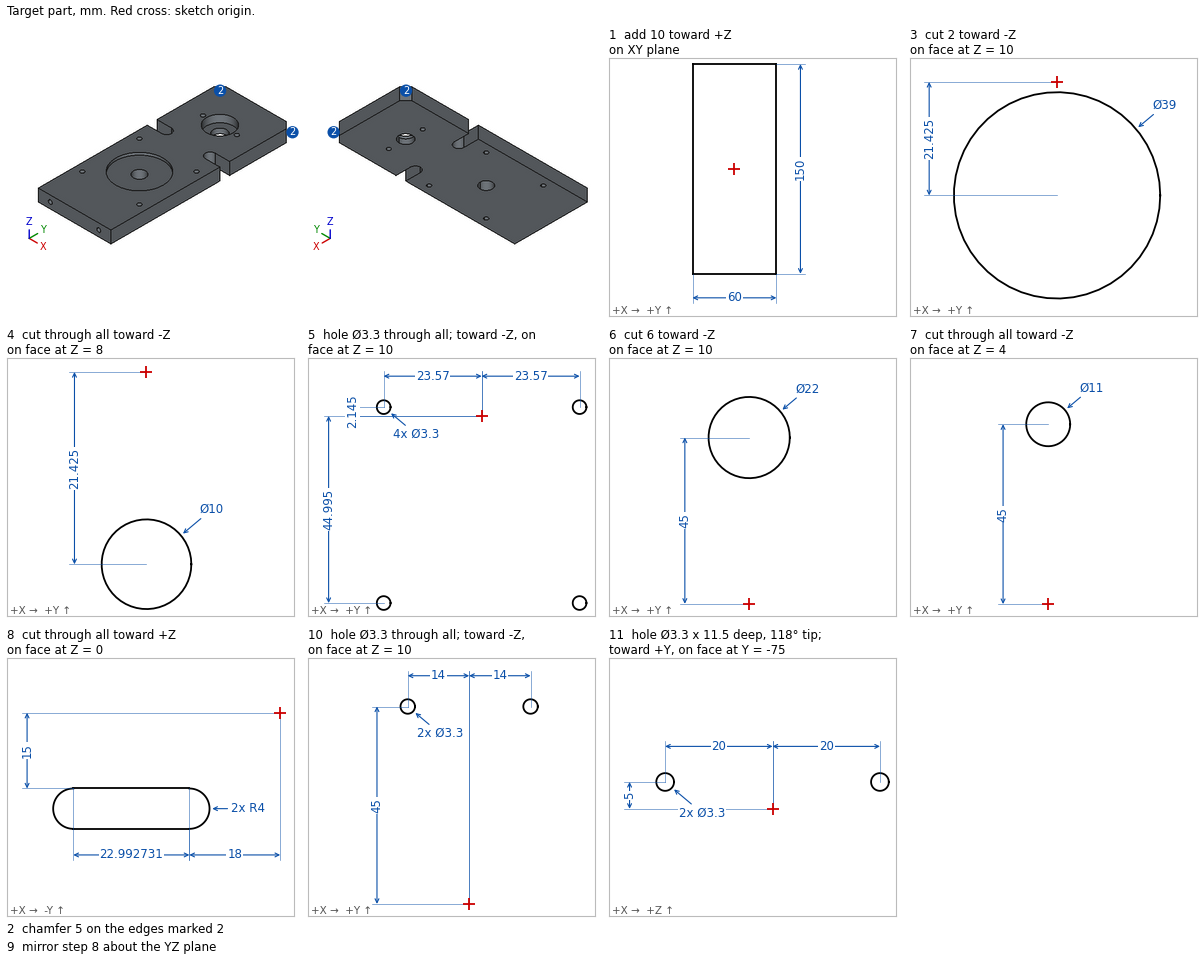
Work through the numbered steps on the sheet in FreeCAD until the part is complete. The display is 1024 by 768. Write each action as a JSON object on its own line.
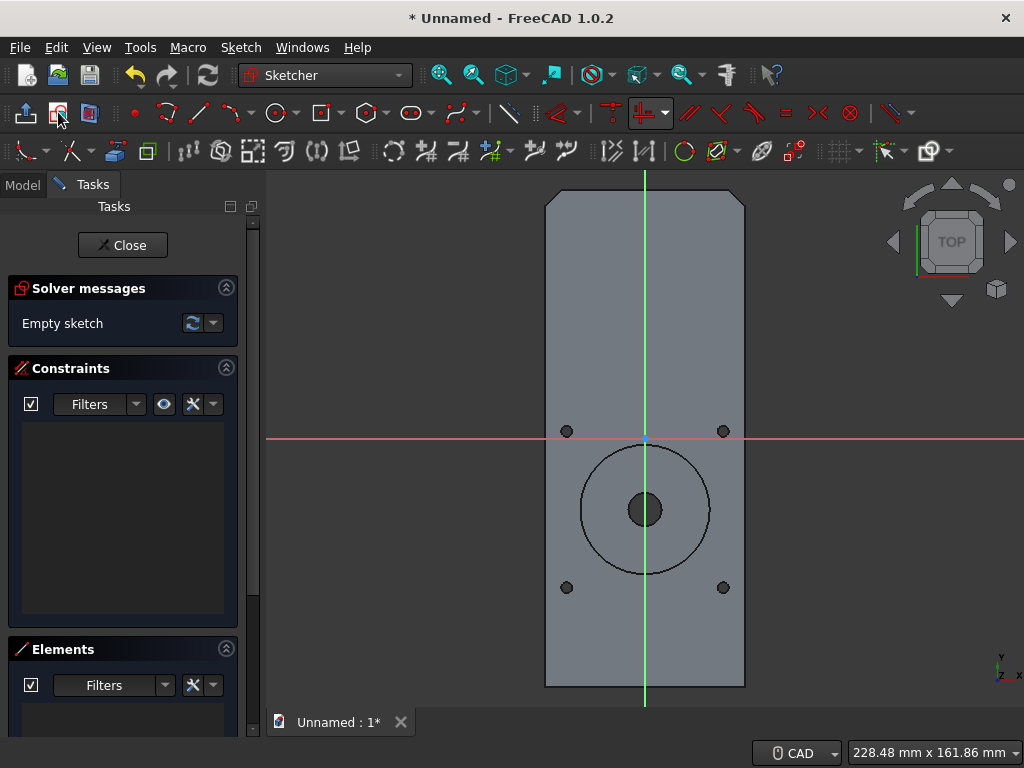
{"action": "scroll", "coordinate": [662, 251], "scroll_direction": "up", "scroll_amount": 8}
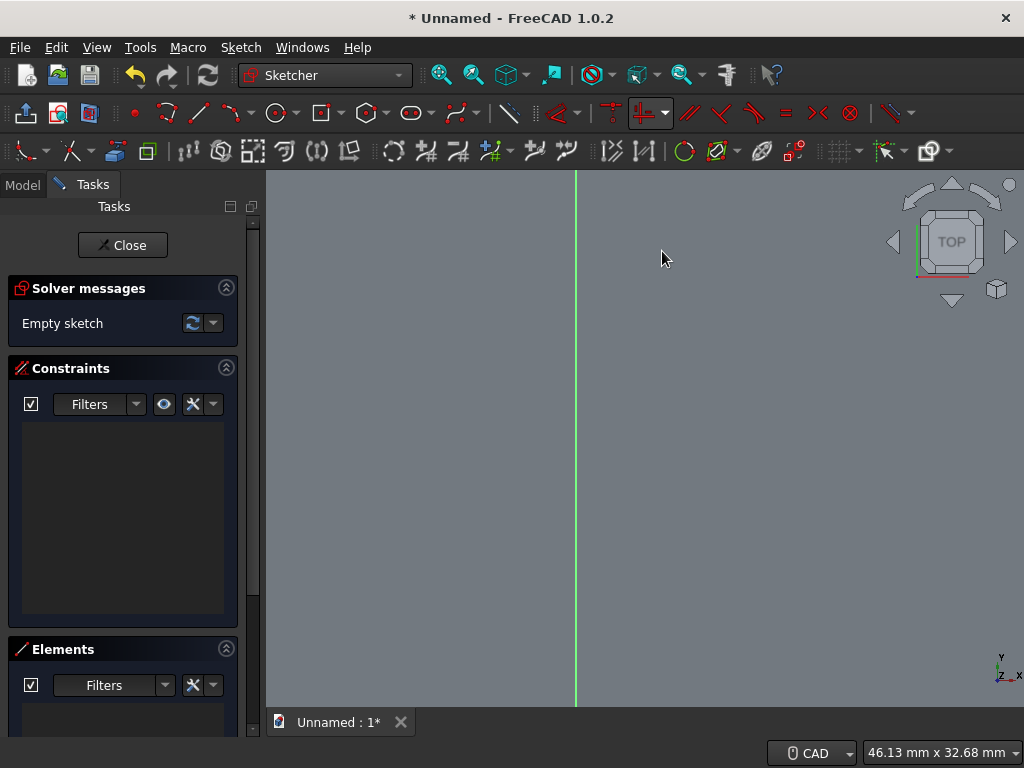
{"action": "key", "text": "g c"}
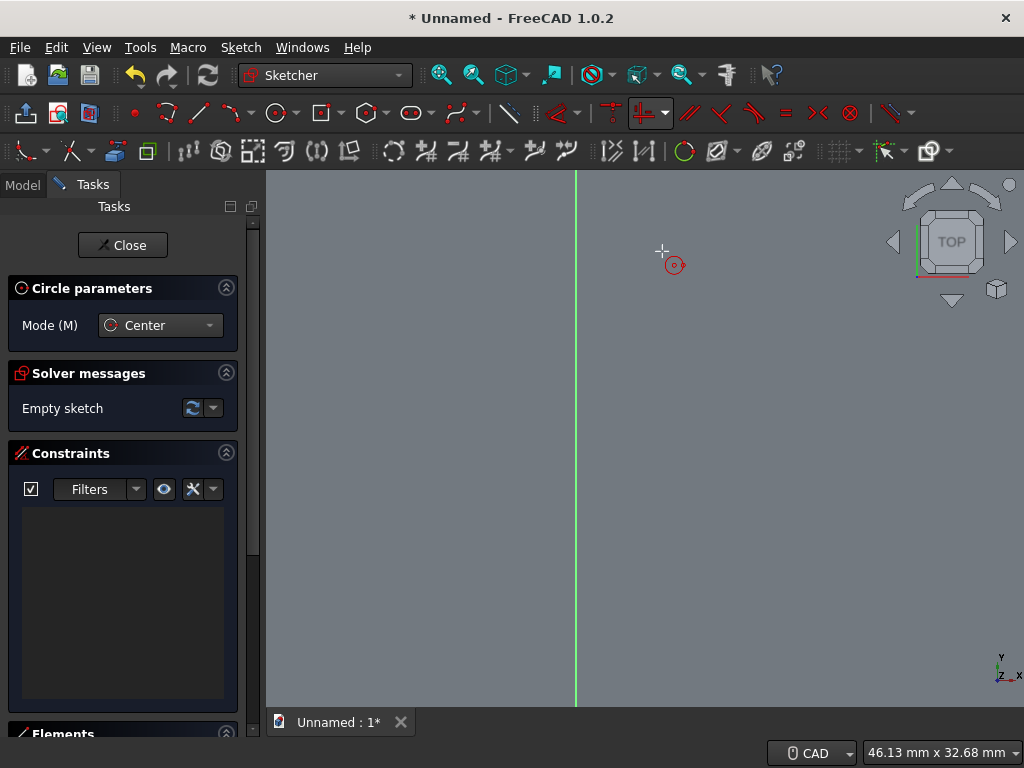
{"action": "left_click", "coordinate": [576, 440]}
{"action": "left_click", "coordinate": [704, 312]}
{"action": "key", "text": "Escape"}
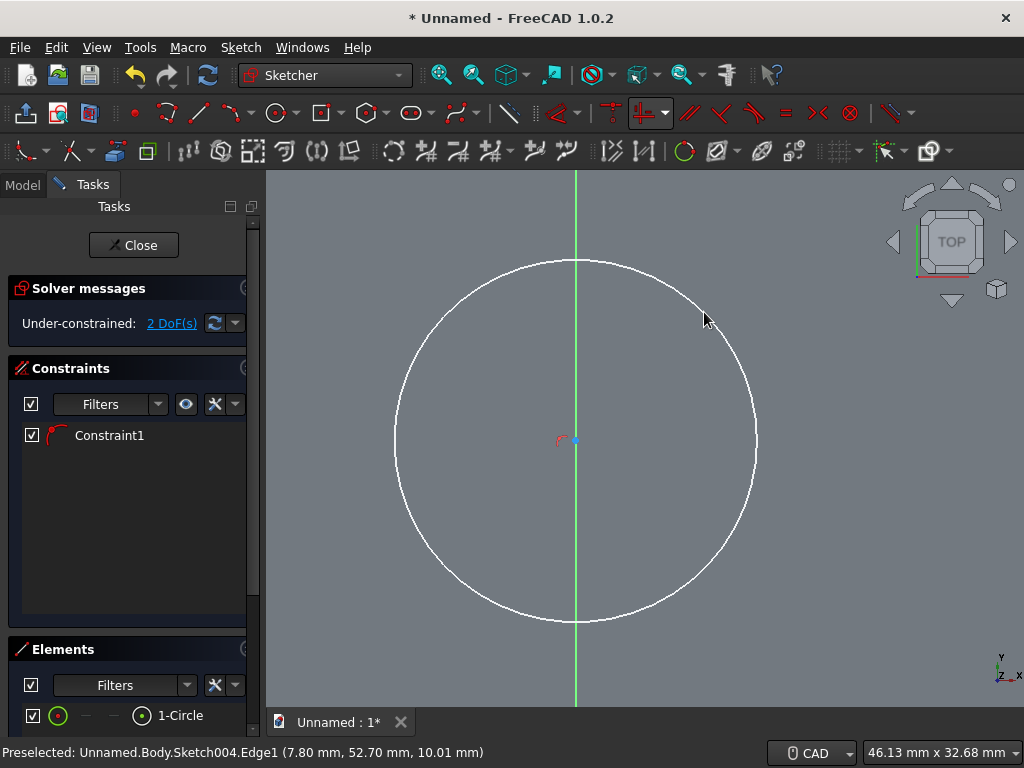
{"action": "left_click", "coordinate": [556, 114]}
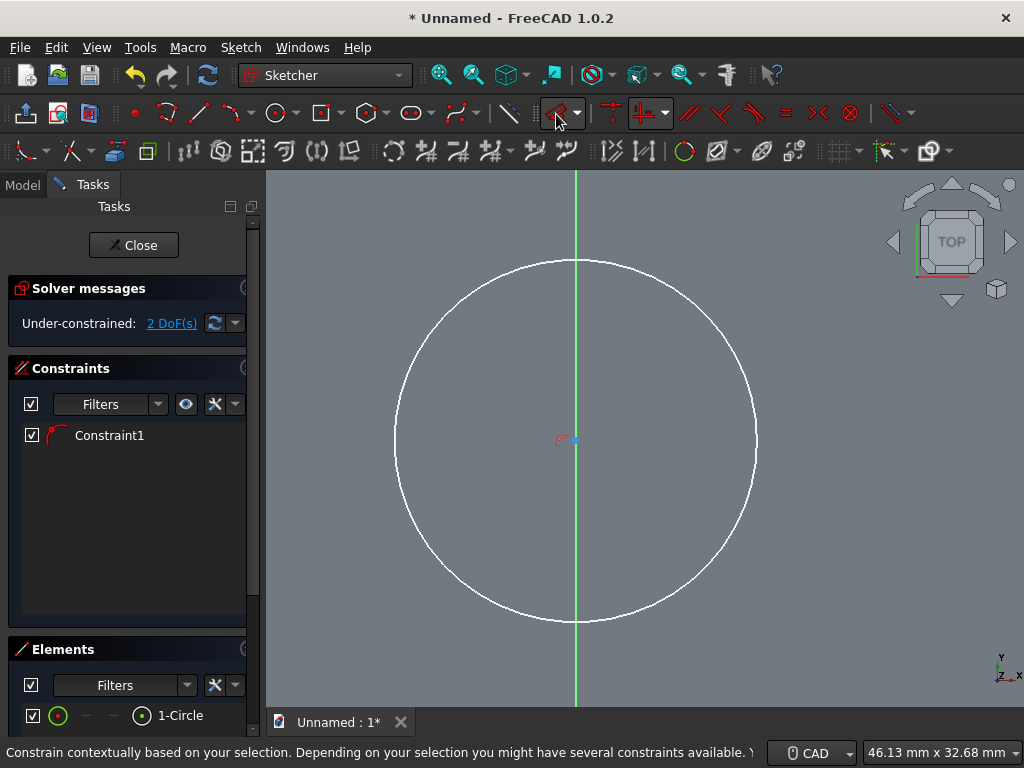
{"action": "left_click", "coordinate": [703, 312]}
{"action": "left_click", "coordinate": [725, 289]}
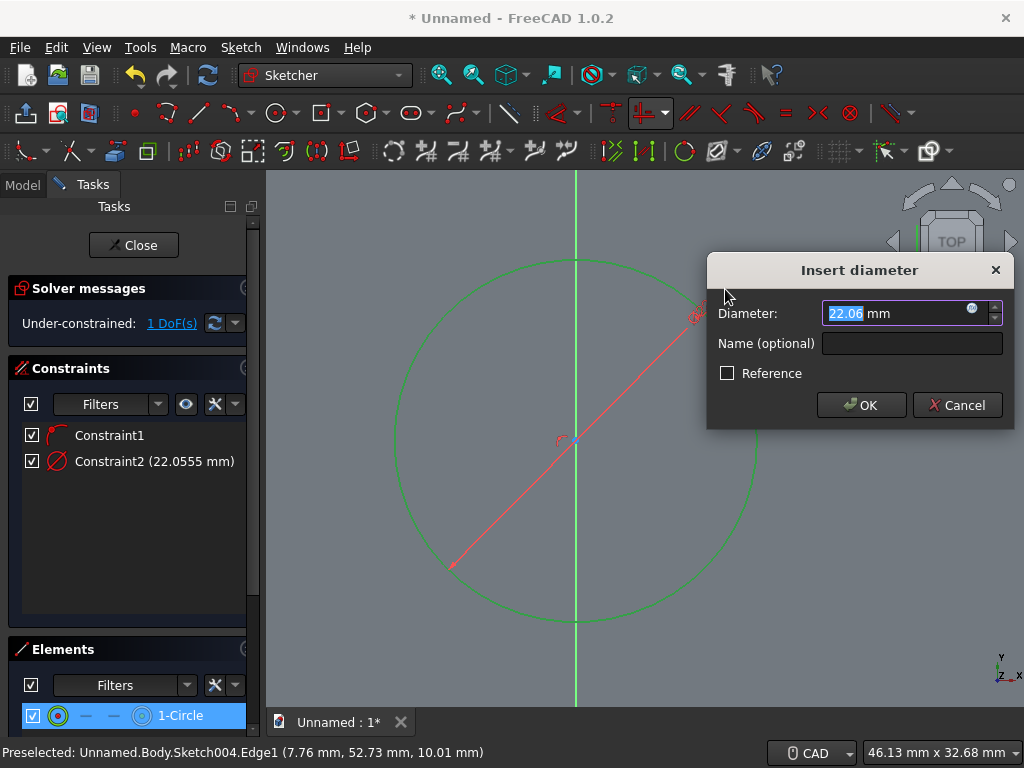
{"action": "type", "text": "22"}
{"action": "key", "text": "Return"}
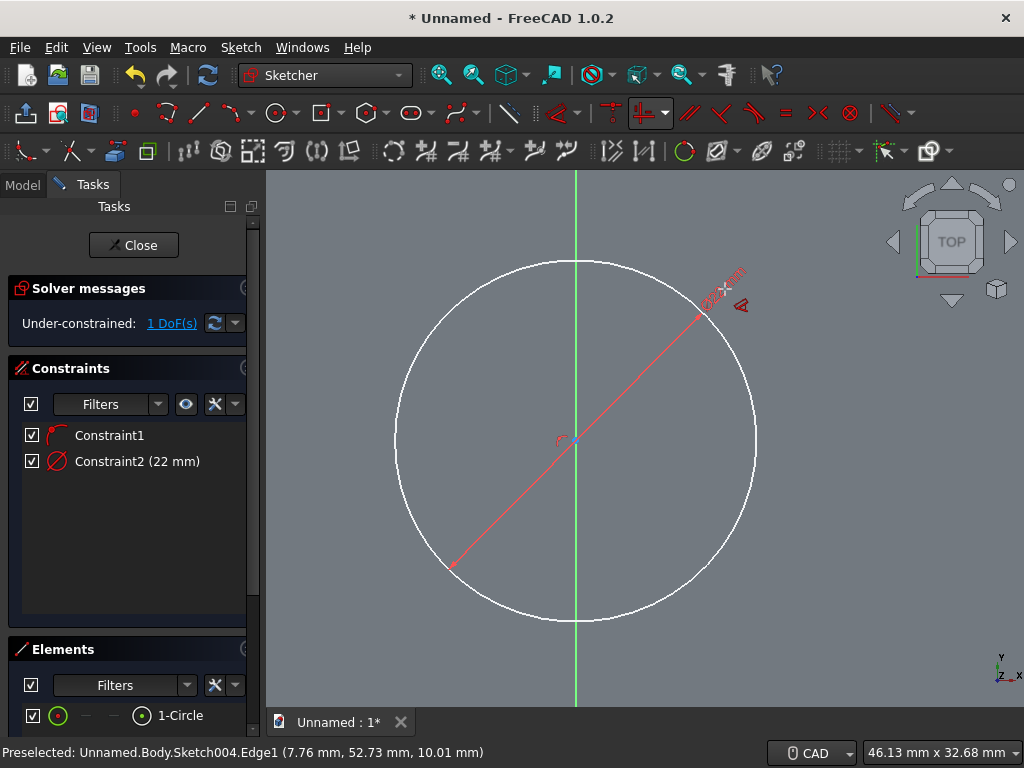
{"action": "left_click", "coordinate": [576, 441]}
{"action": "left_click", "coordinate": [610, 560]}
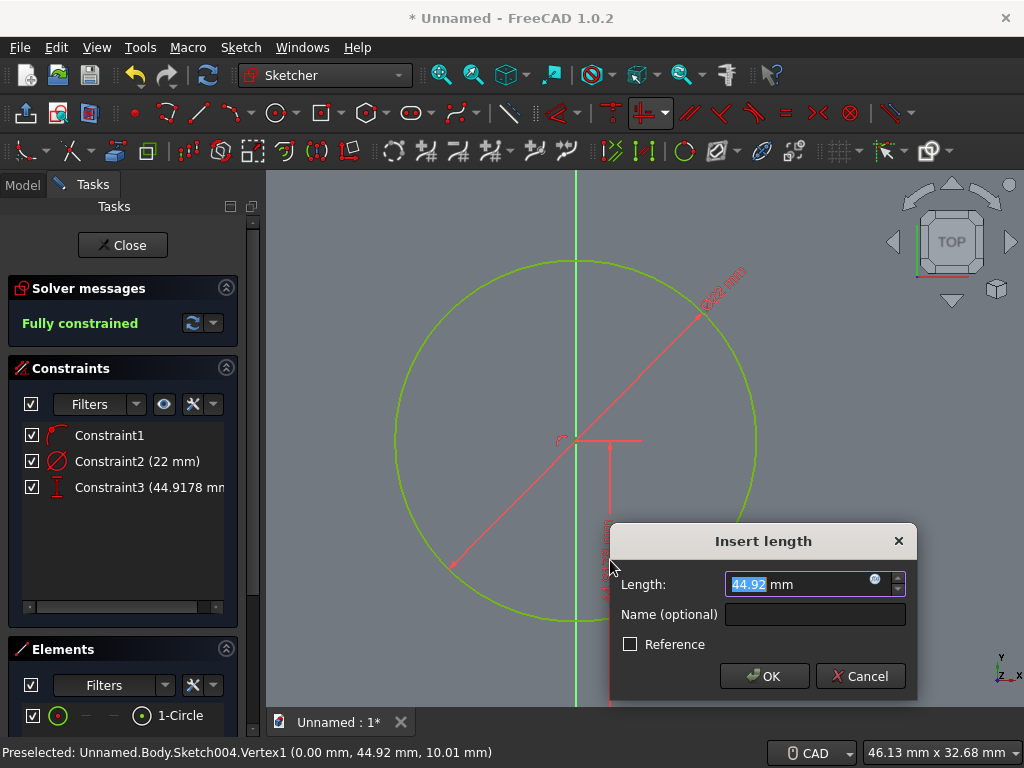
{"action": "type", "text": "45"}
{"action": "key", "text": "Return"}
{"action": "key", "text": "Escape"}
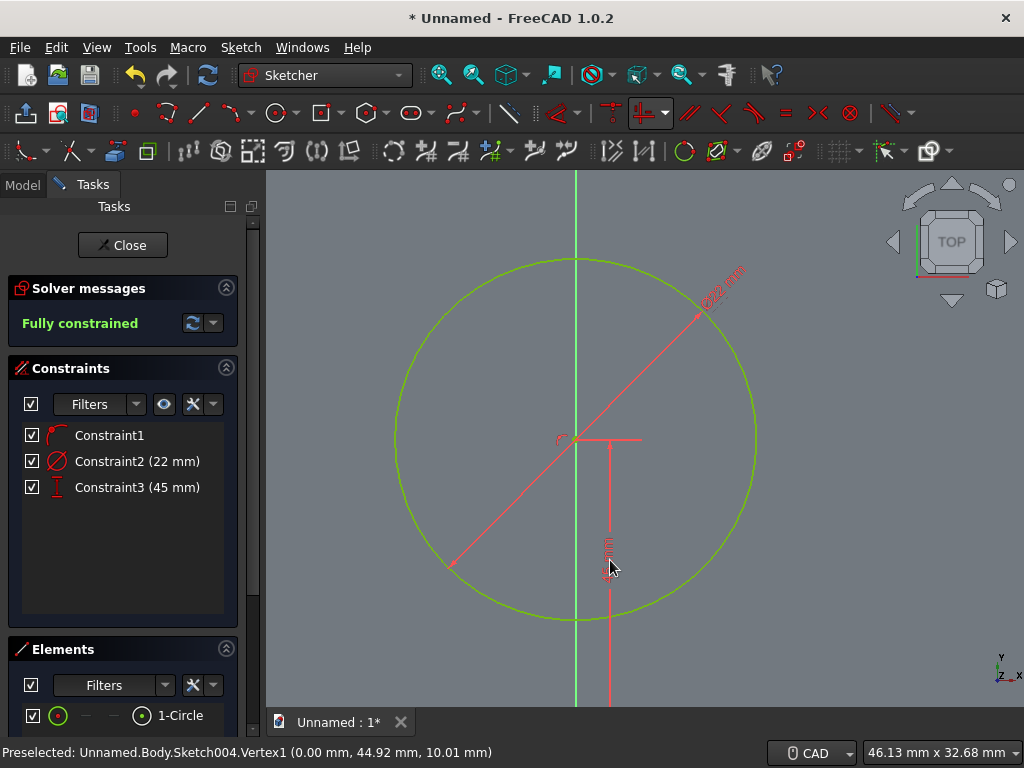
{"action": "left_click", "coordinate": [123, 245]}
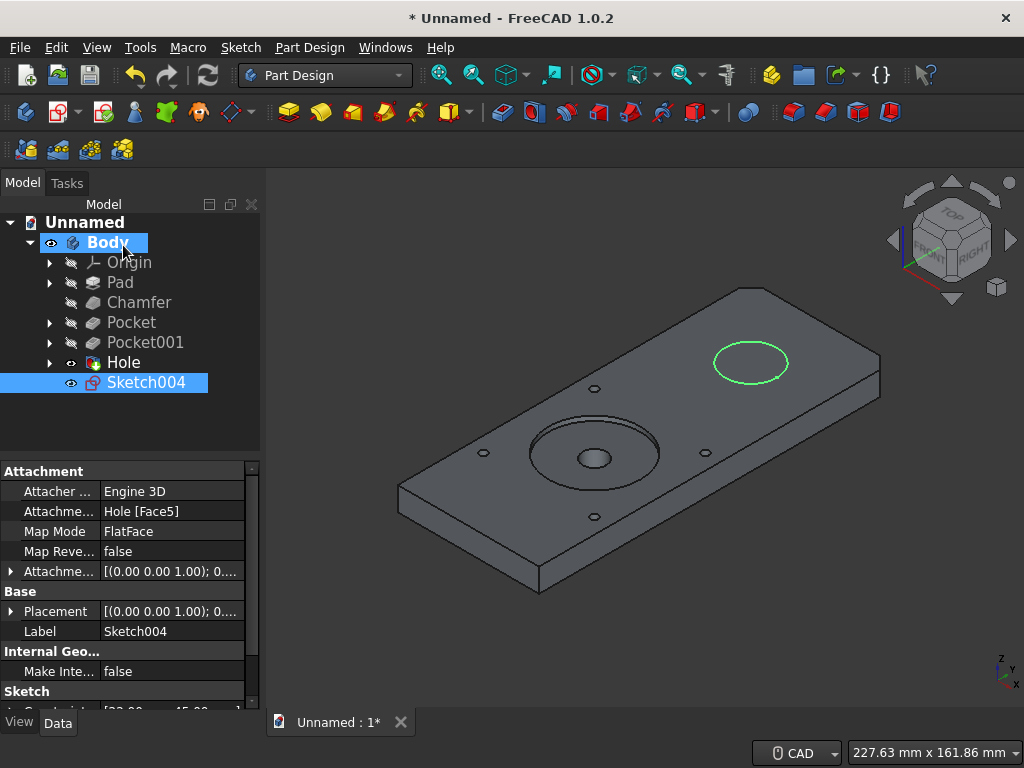
{"action": "left_click", "coordinate": [504, 112]}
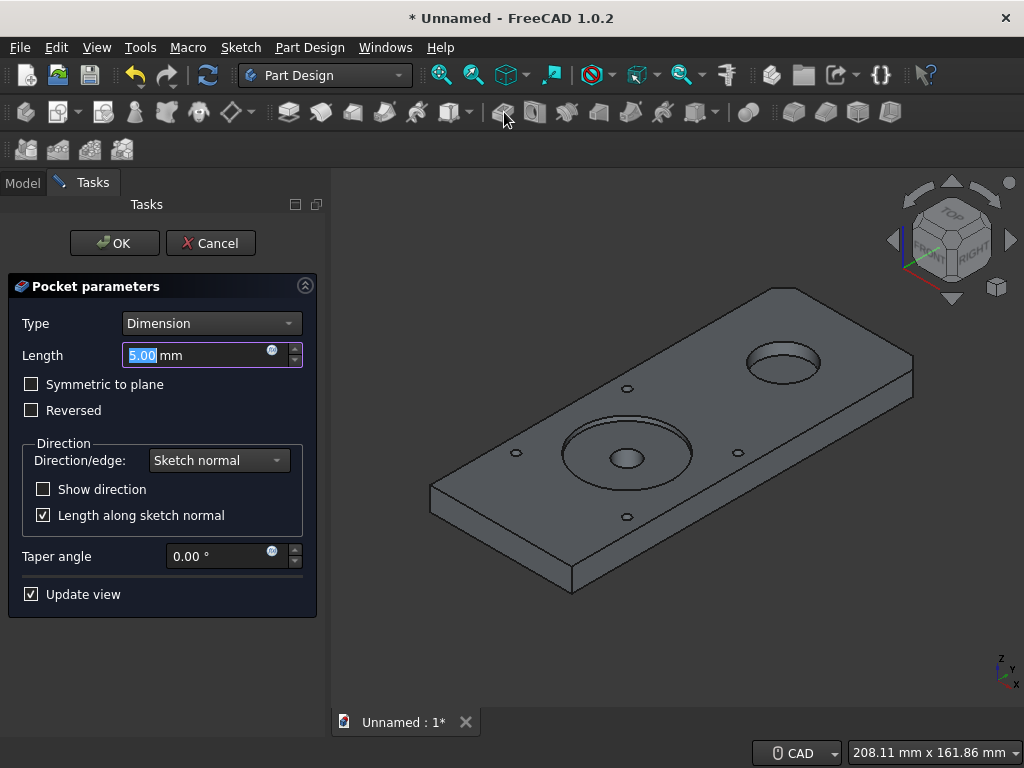
{"action": "type", "text": "6"}
{"action": "key", "text": "Tab"}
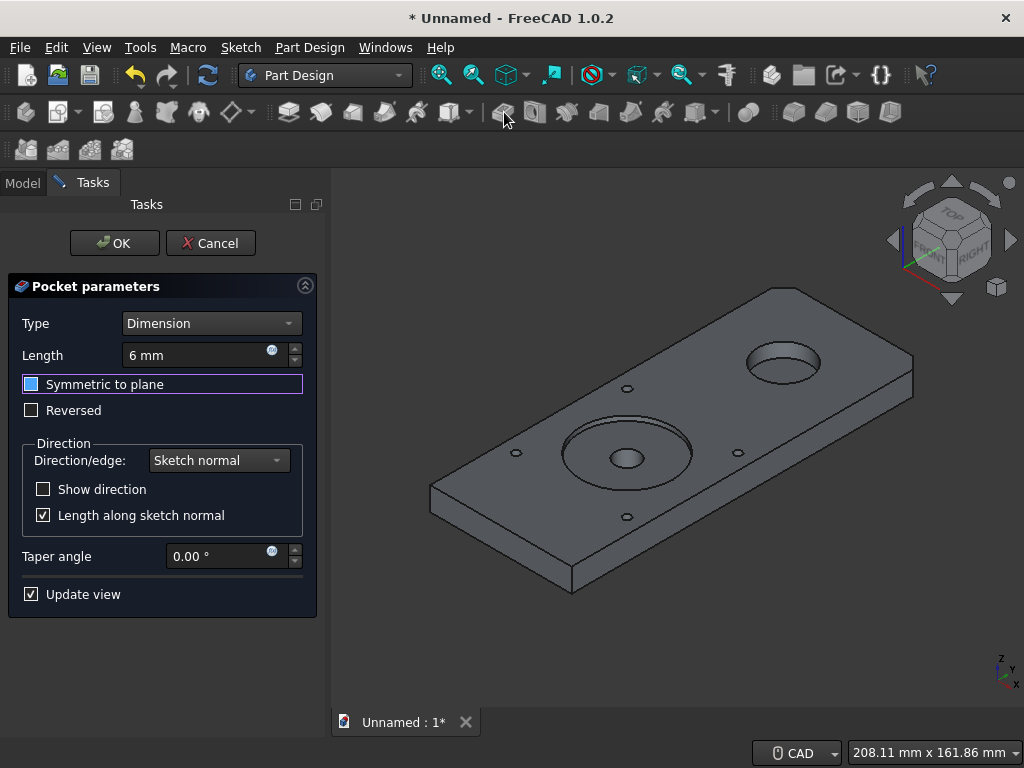
{"action": "left_click", "coordinate": [115, 243]}